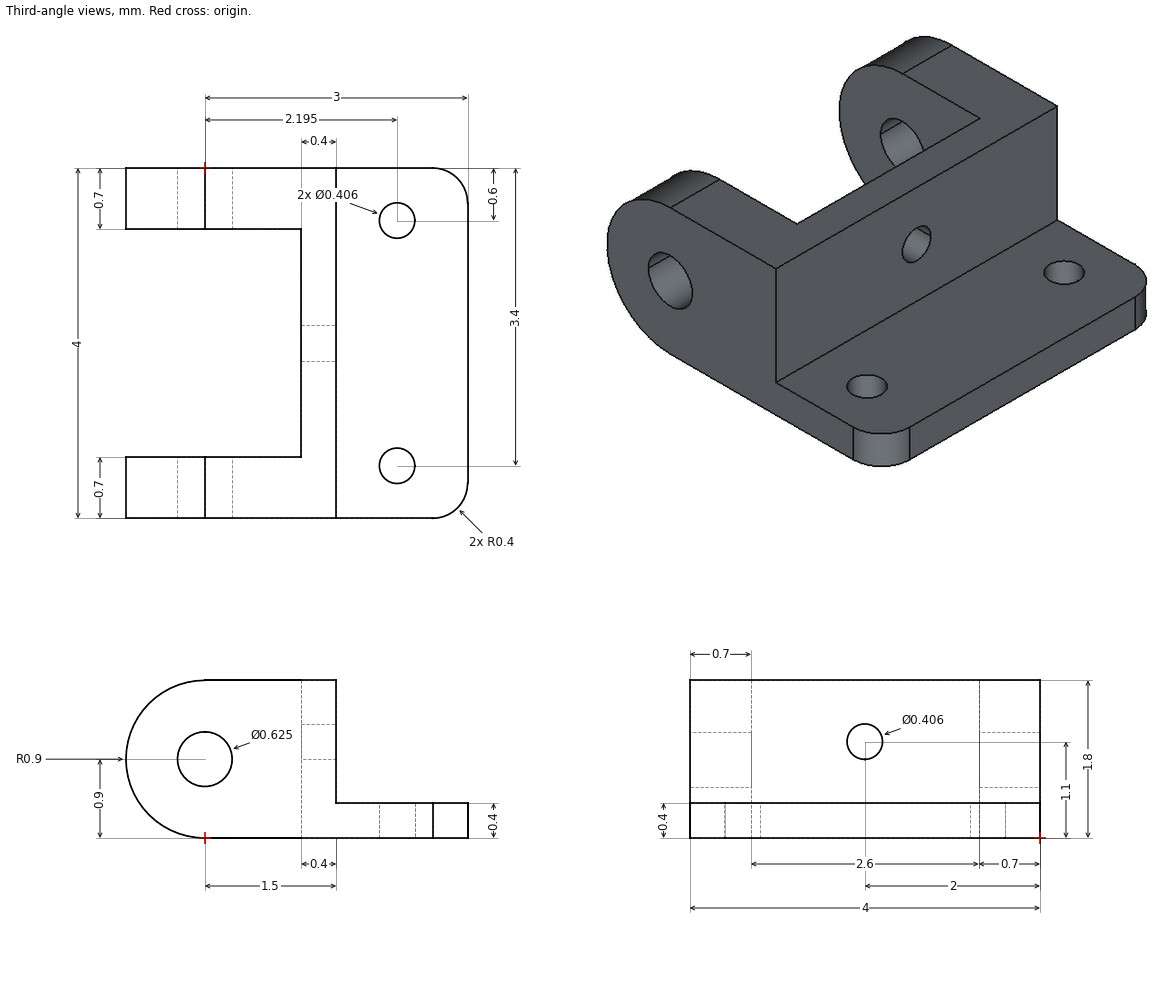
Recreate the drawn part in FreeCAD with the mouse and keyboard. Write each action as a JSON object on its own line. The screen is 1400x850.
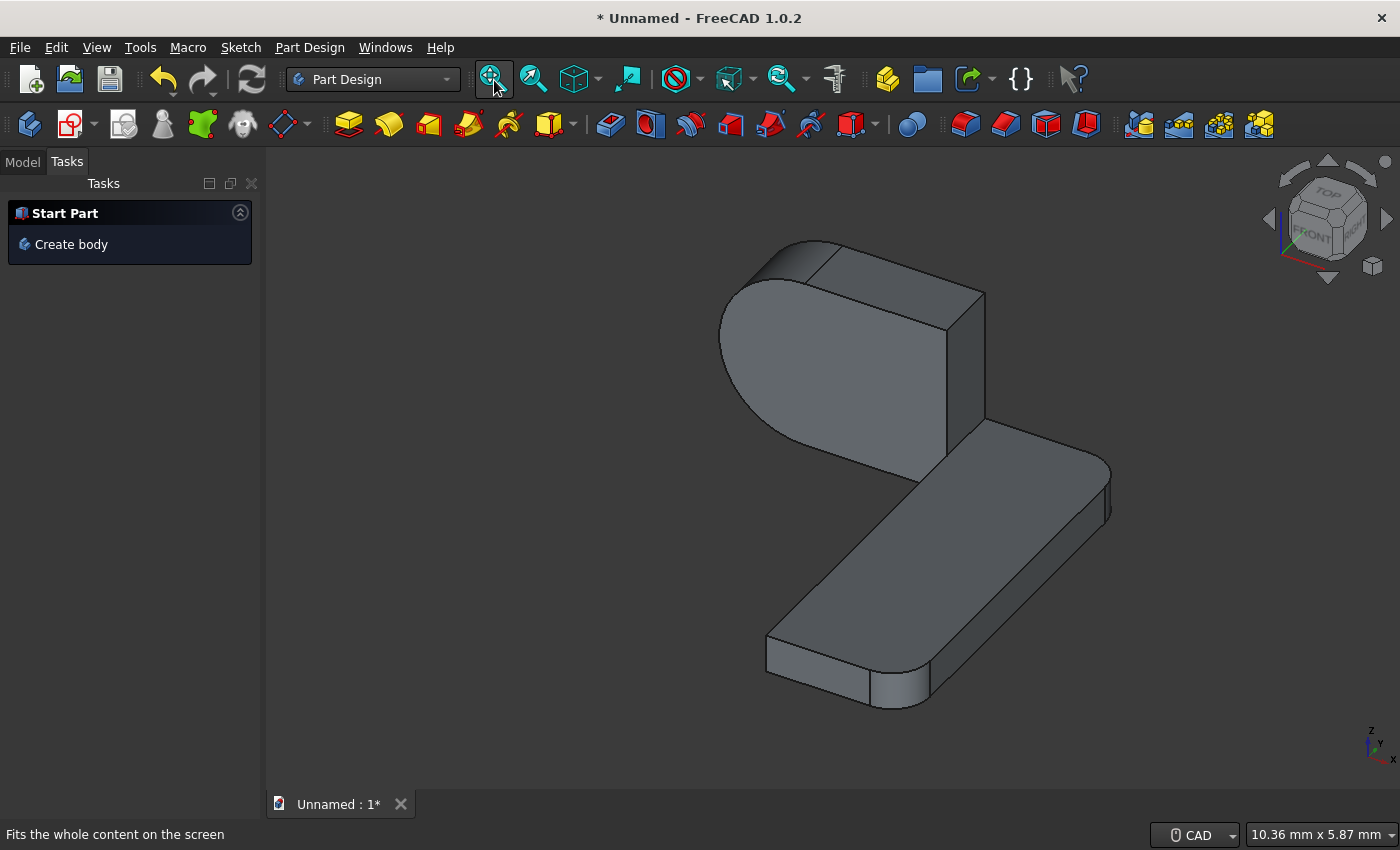
{"action": "left_click", "coordinate": [23, 161]}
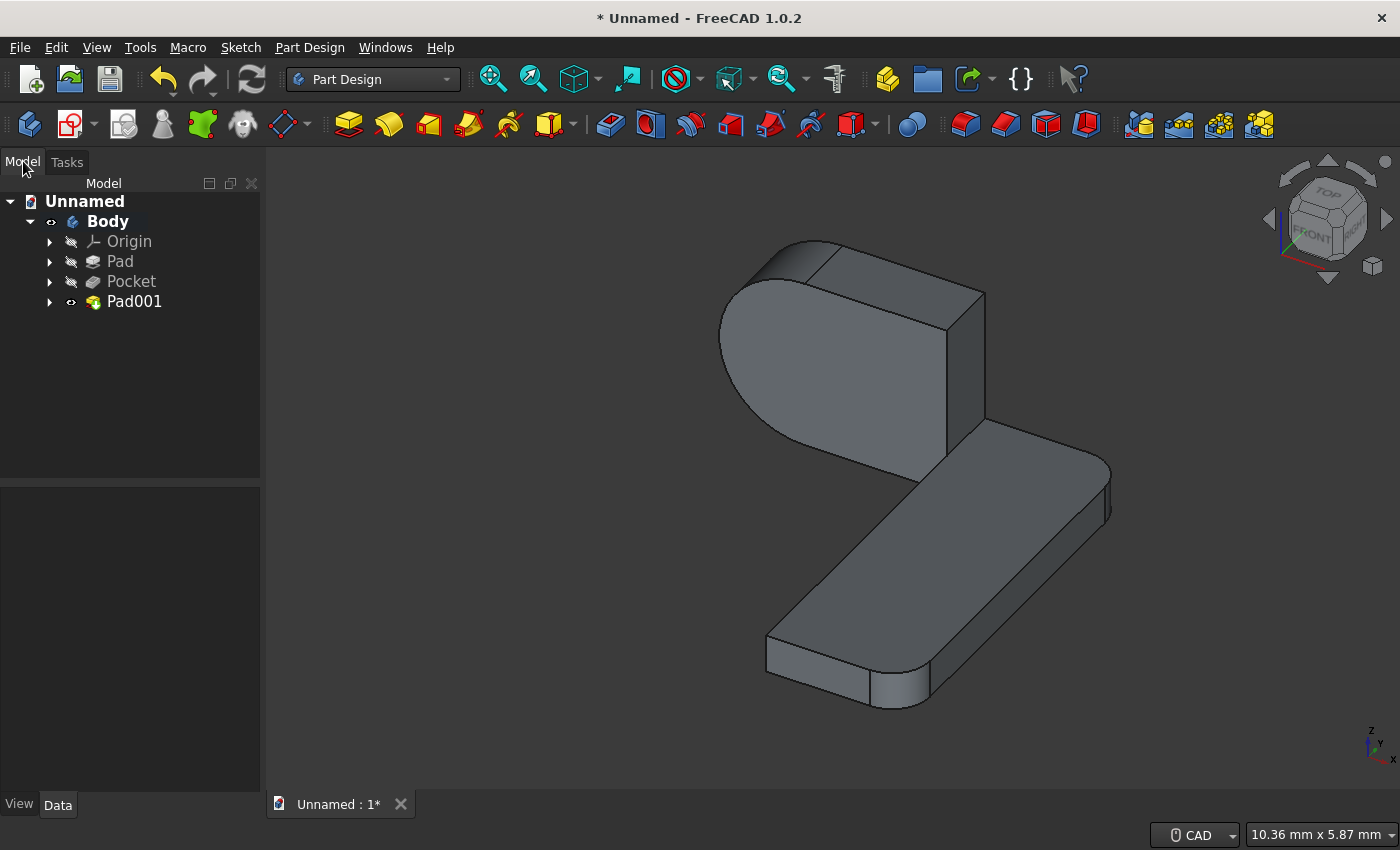
{"action": "left_click", "coordinate": [50, 242]}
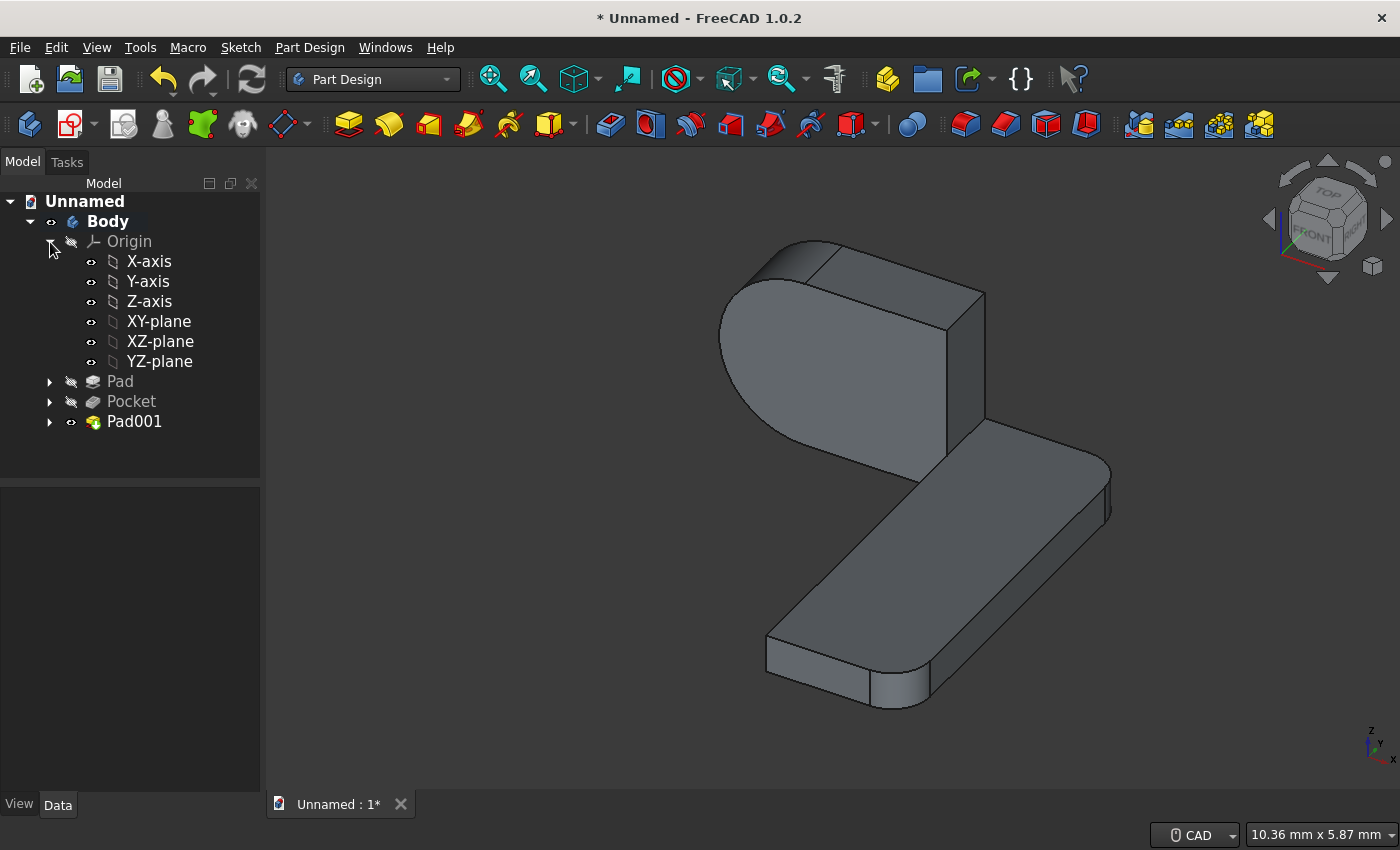
{"action": "left_click", "coordinate": [136, 342]}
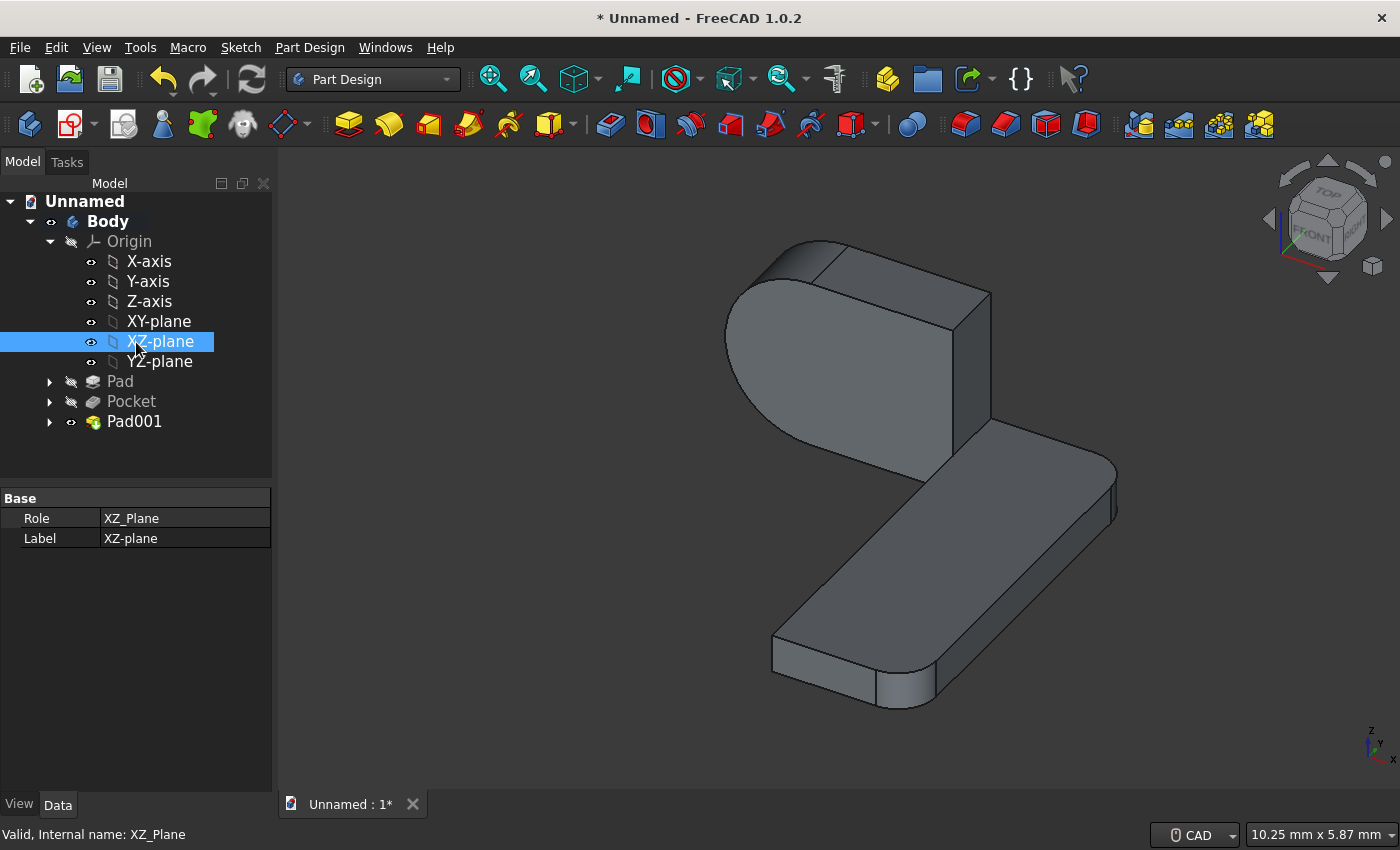
{"action": "left_click", "coordinate": [284, 124]}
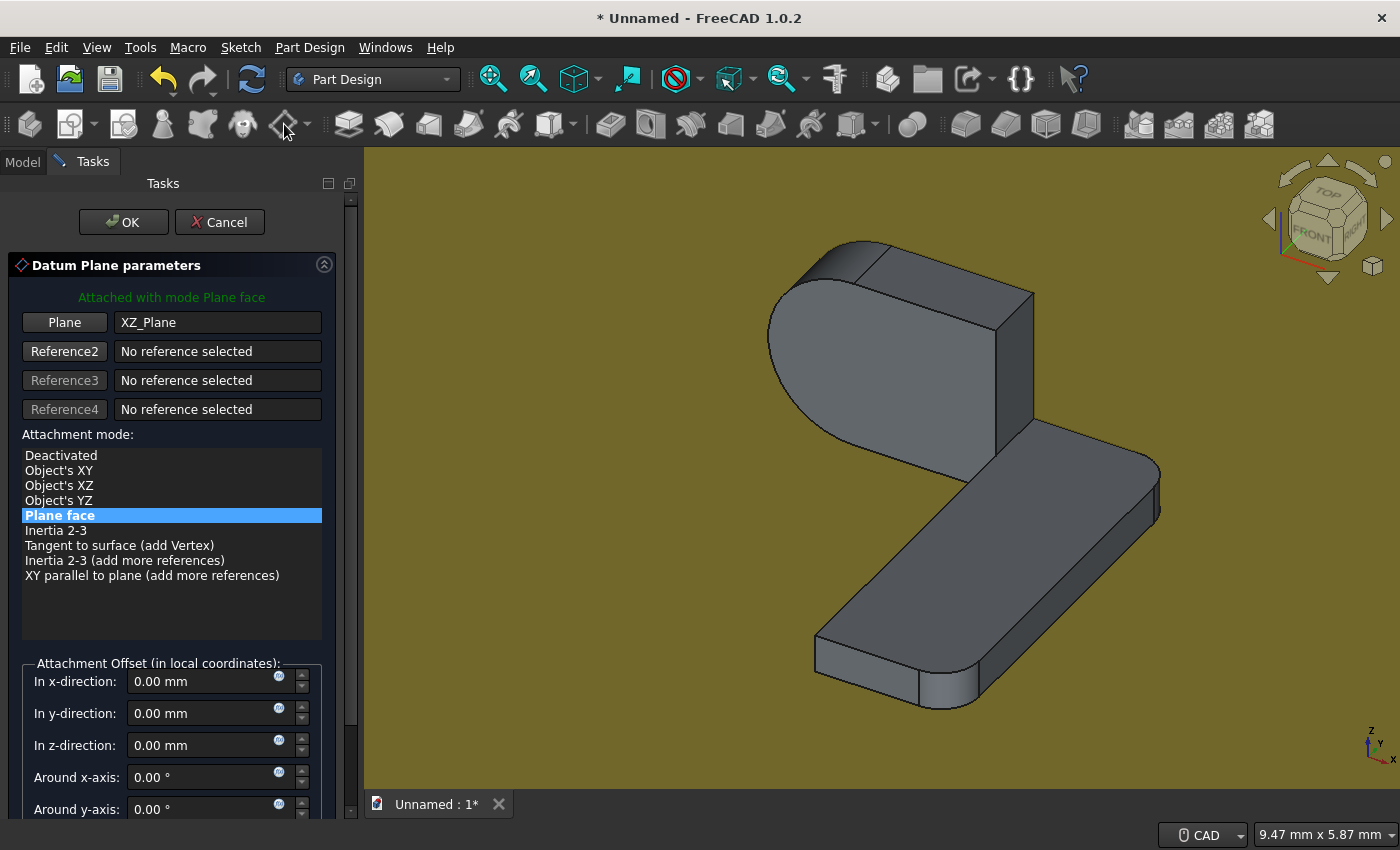
{"action": "triple_click", "coordinate": [210, 745]}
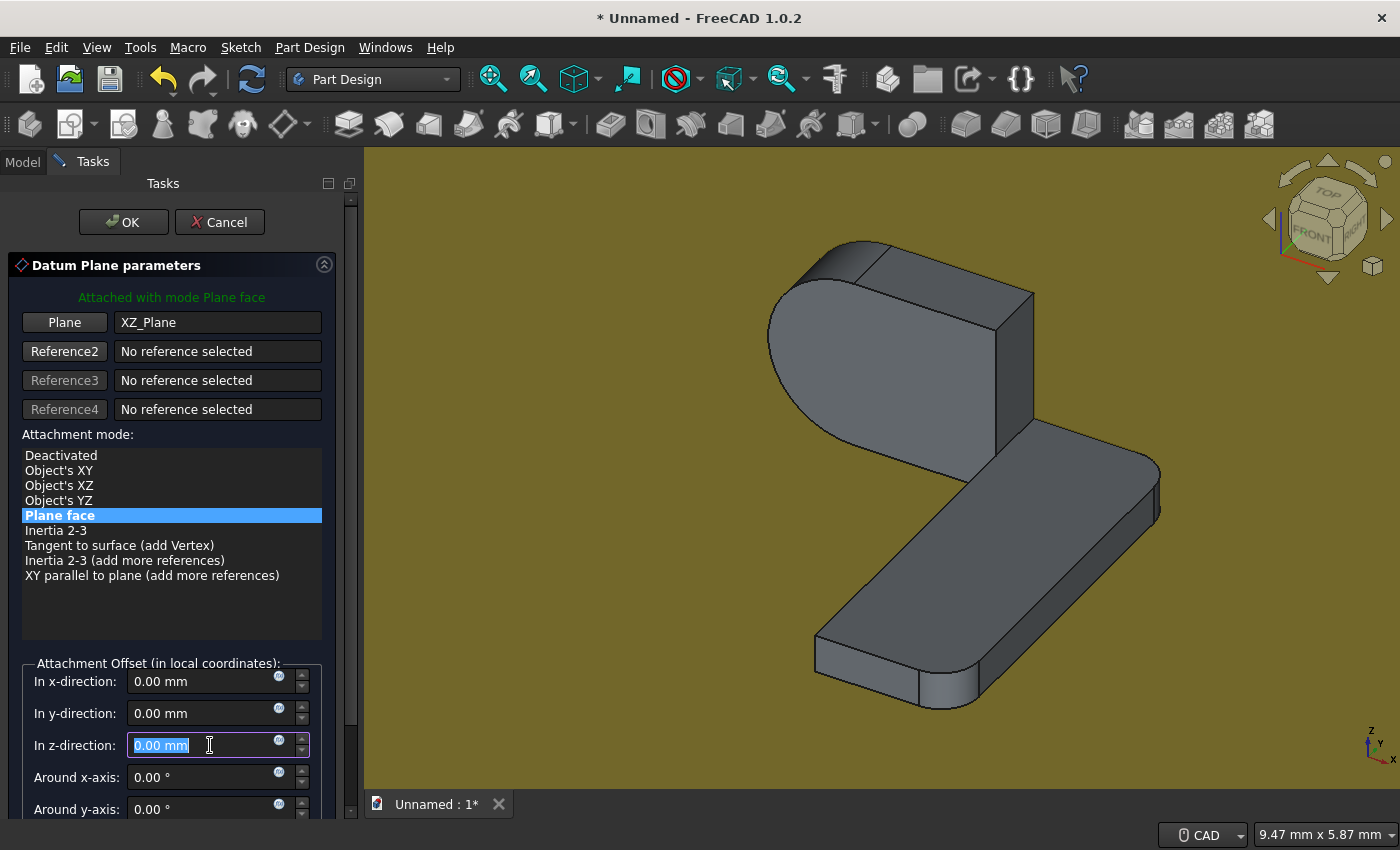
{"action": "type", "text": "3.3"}
{"action": "key", "text": "Tab"}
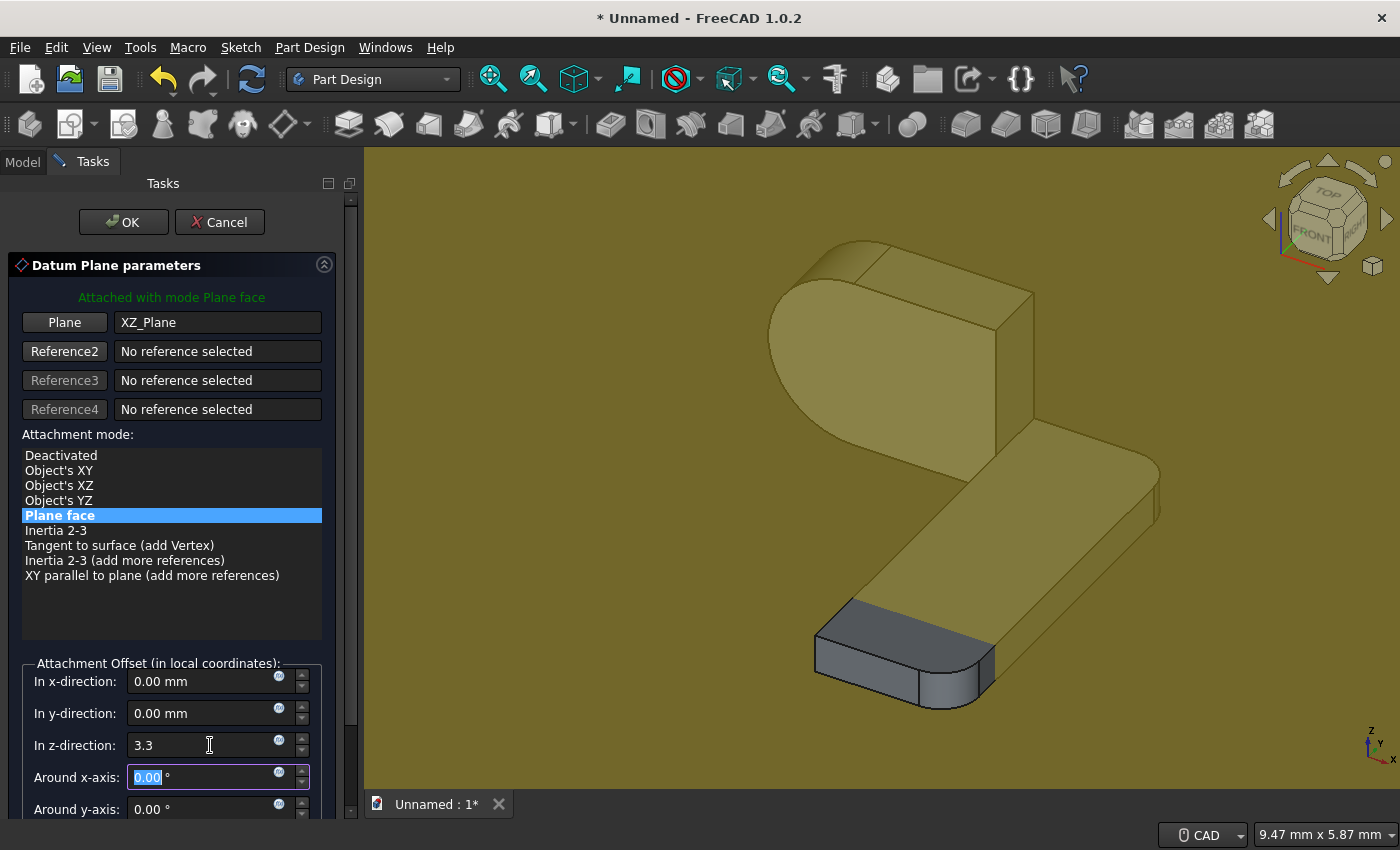
{"action": "left_click", "coordinate": [124, 222]}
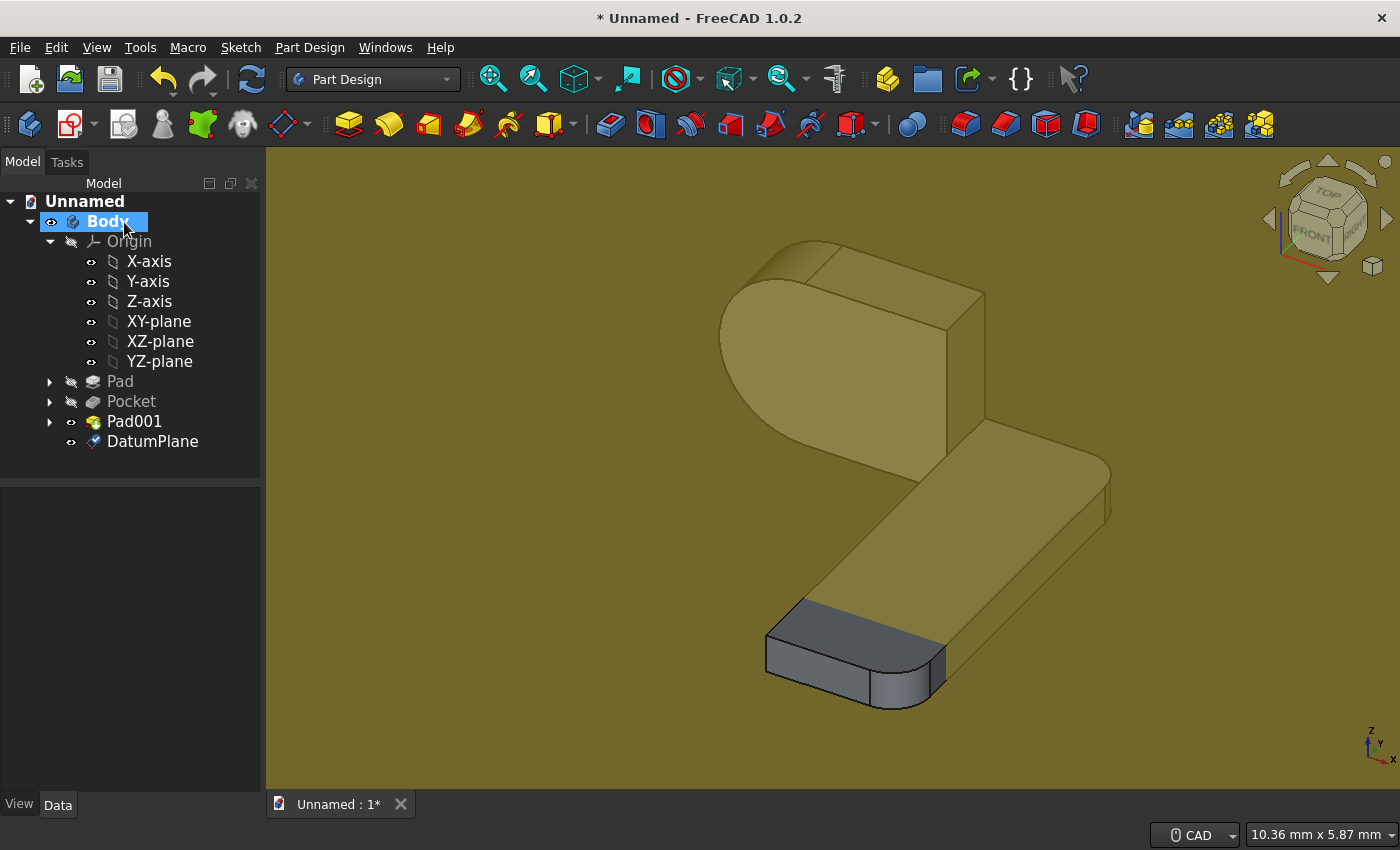
{"action": "left_click", "coordinate": [116, 442]}